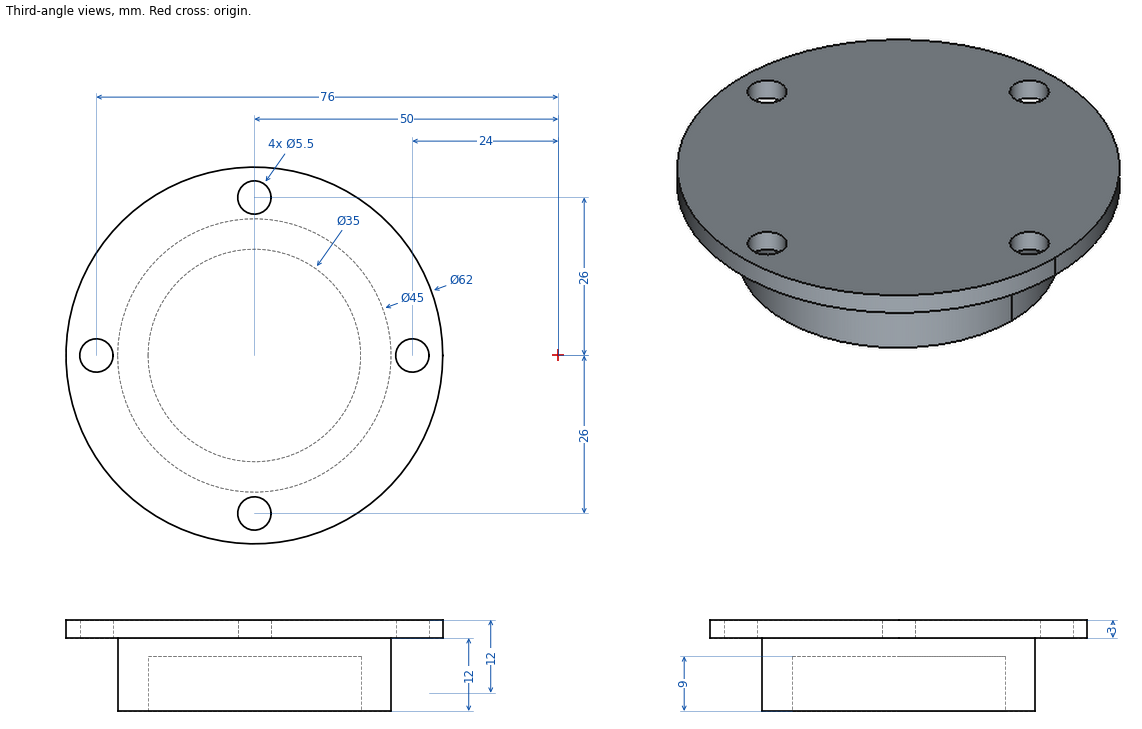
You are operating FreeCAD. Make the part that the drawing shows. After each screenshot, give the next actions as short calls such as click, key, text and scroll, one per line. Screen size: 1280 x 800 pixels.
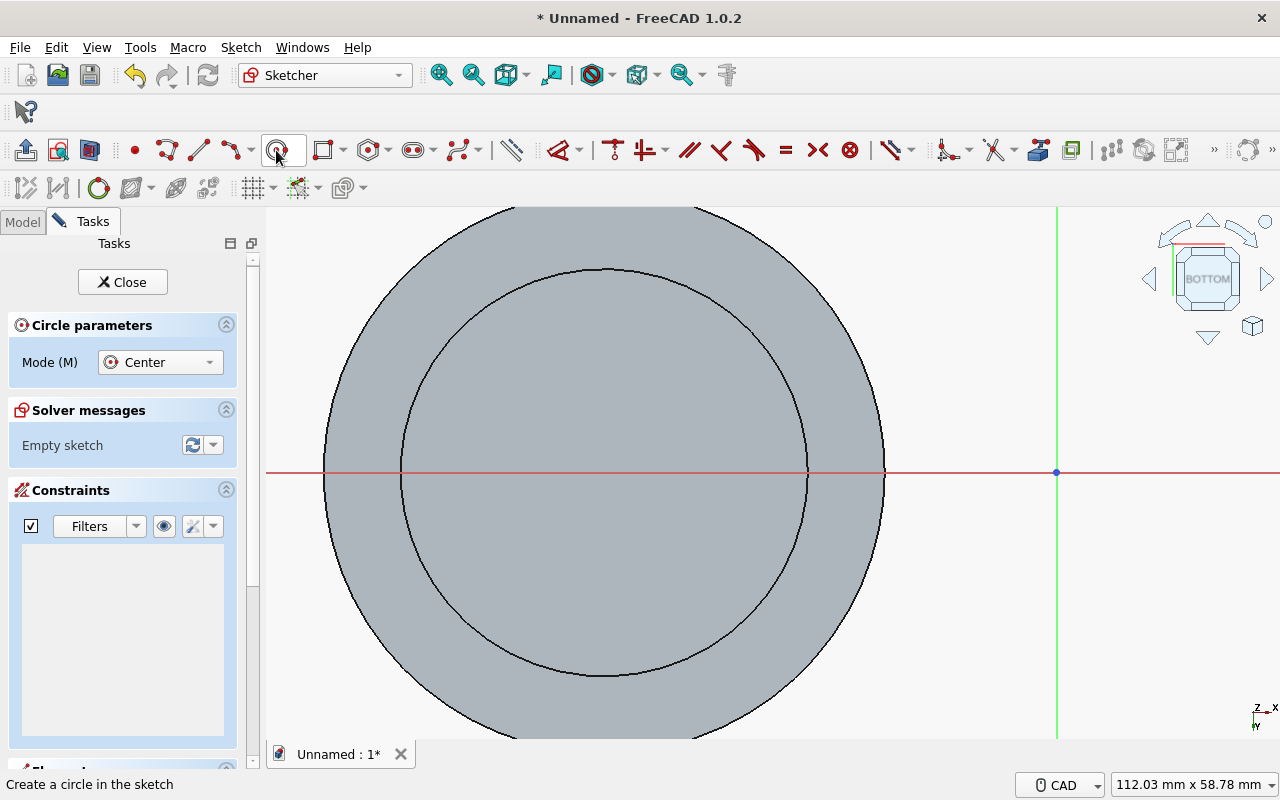
click(604, 473)
move(716, 361)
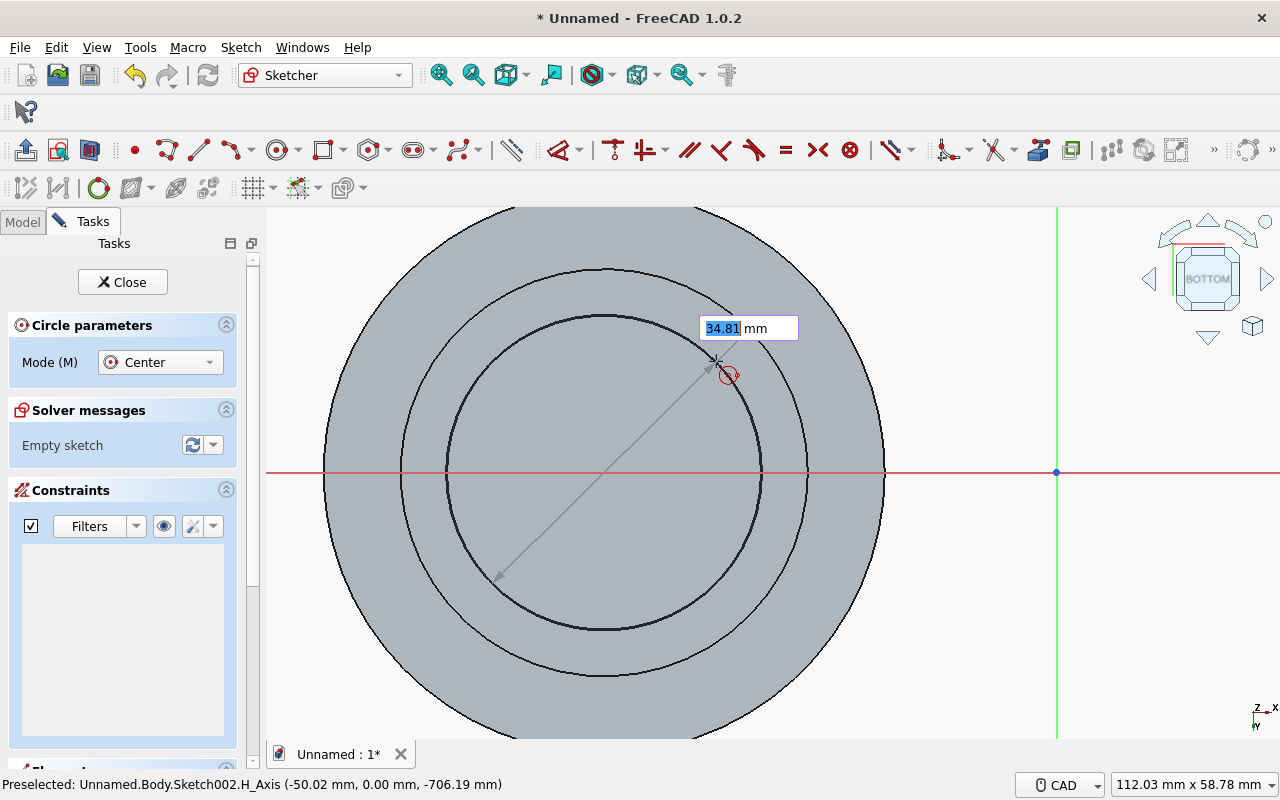
text(35)
key(Return)
key(Escape)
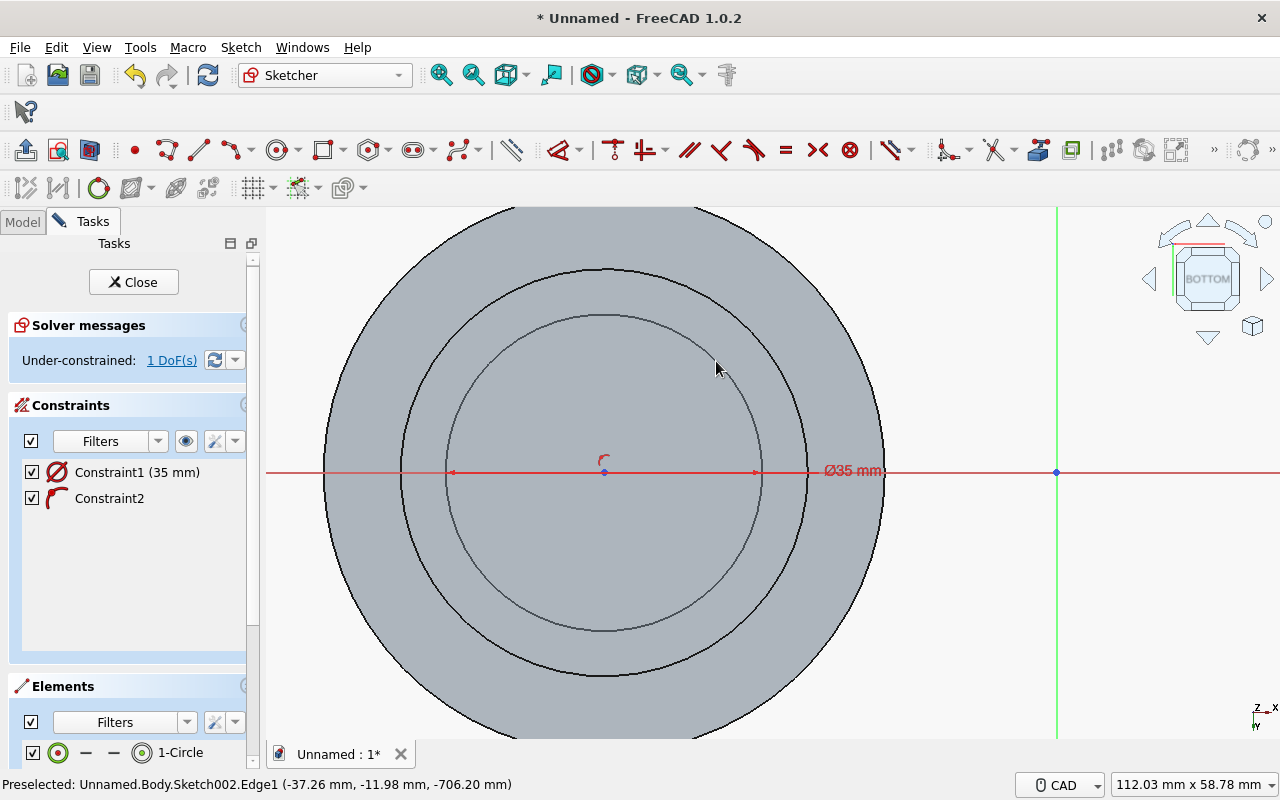
click(558, 150)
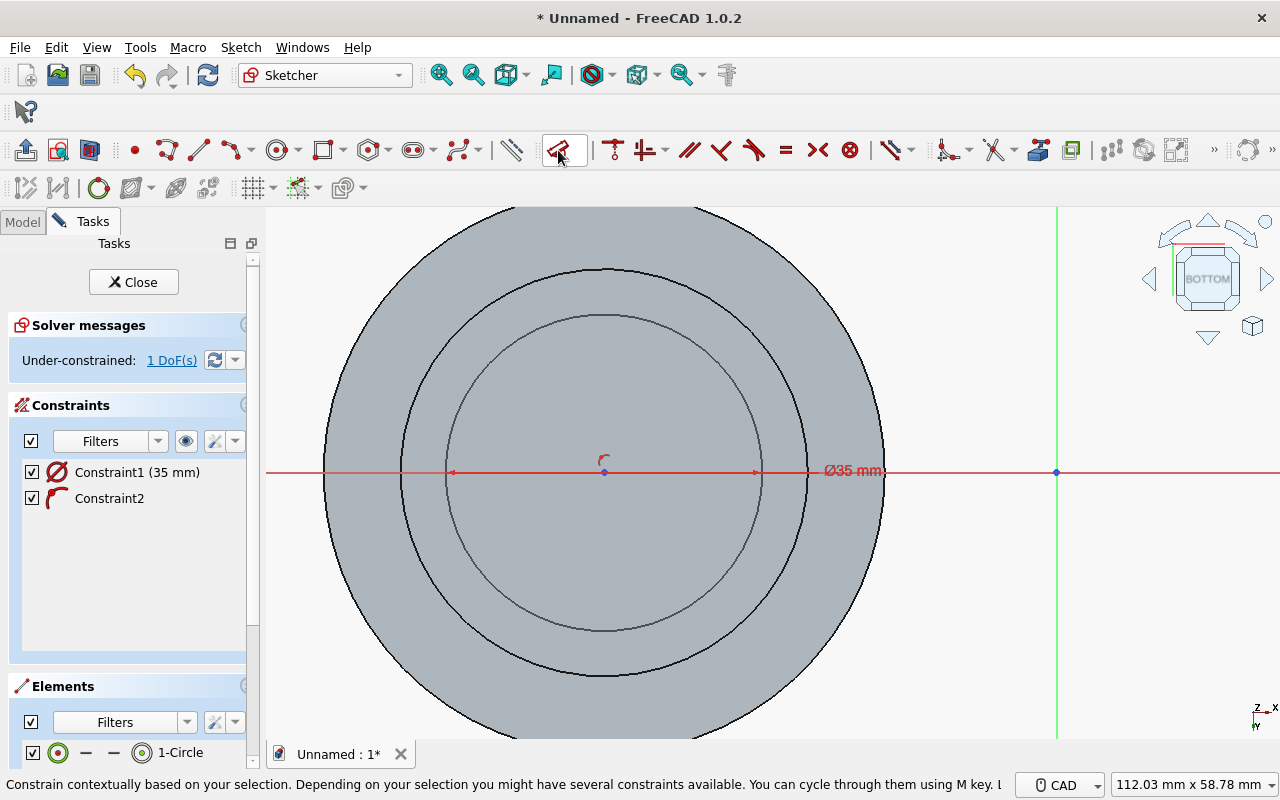
click(604, 473)
click(830, 507)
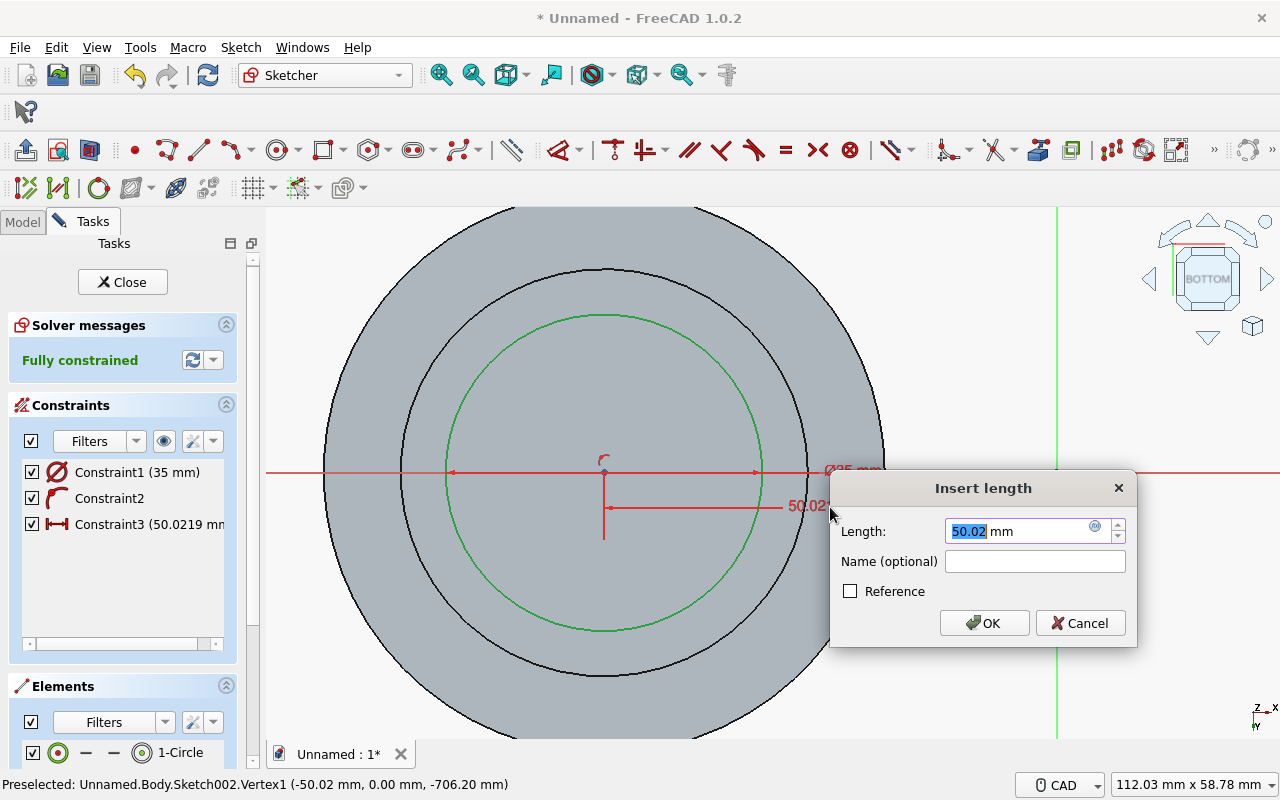
text(50)
key(Return)
key(Escape)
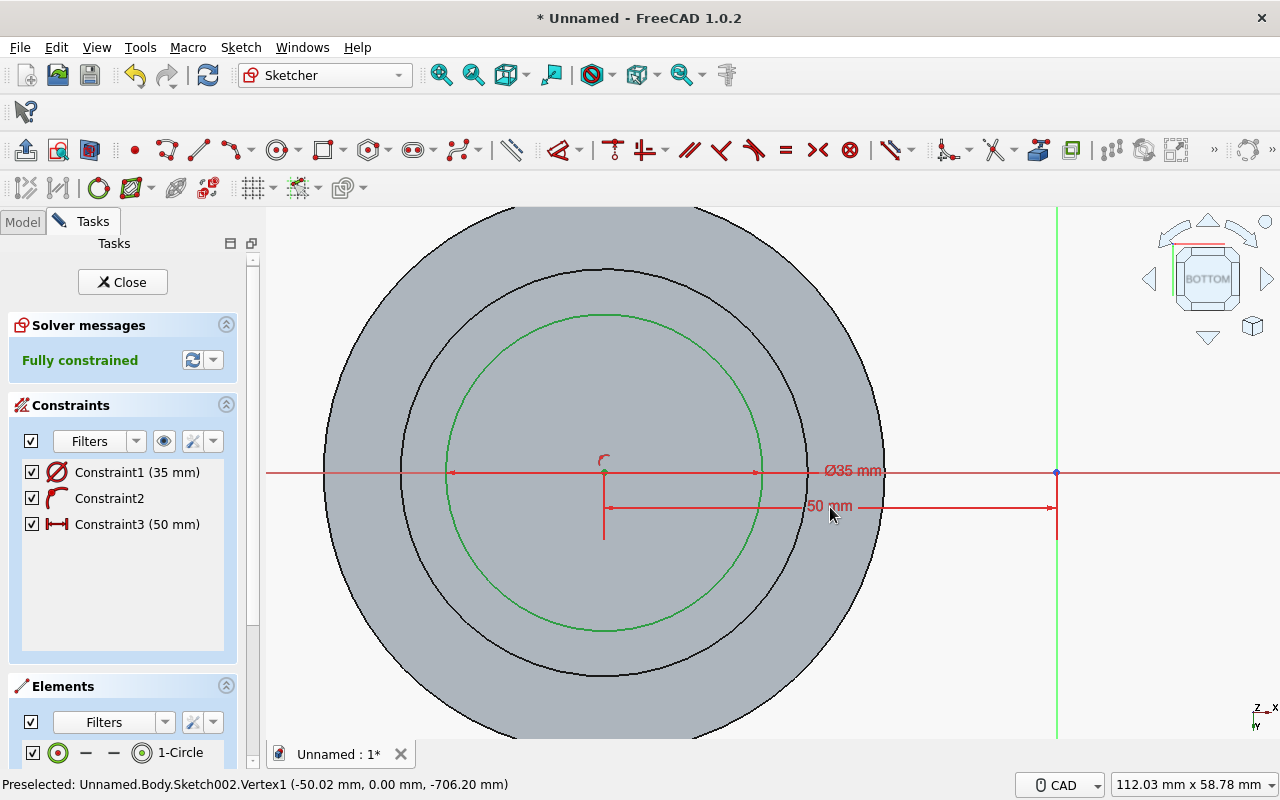
click(123, 282)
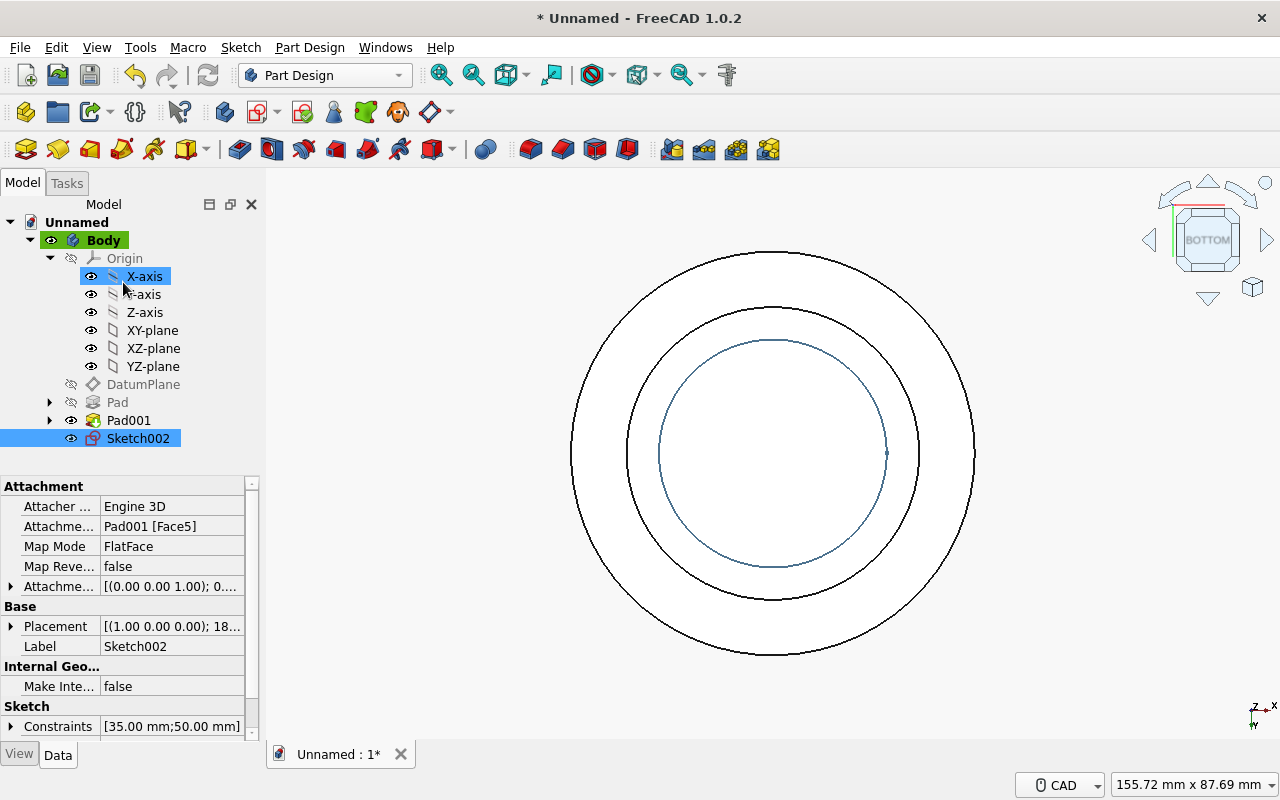
click(240, 150)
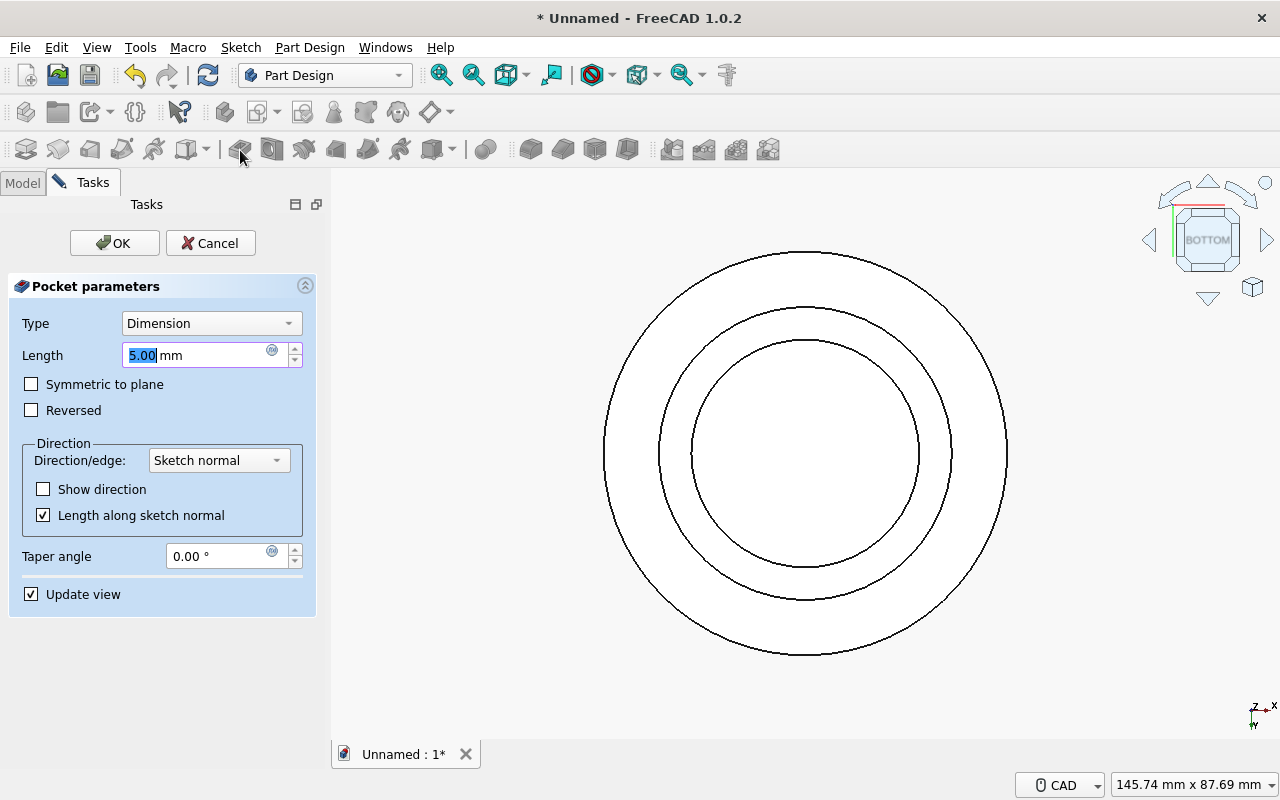
text(9)
key(Tab)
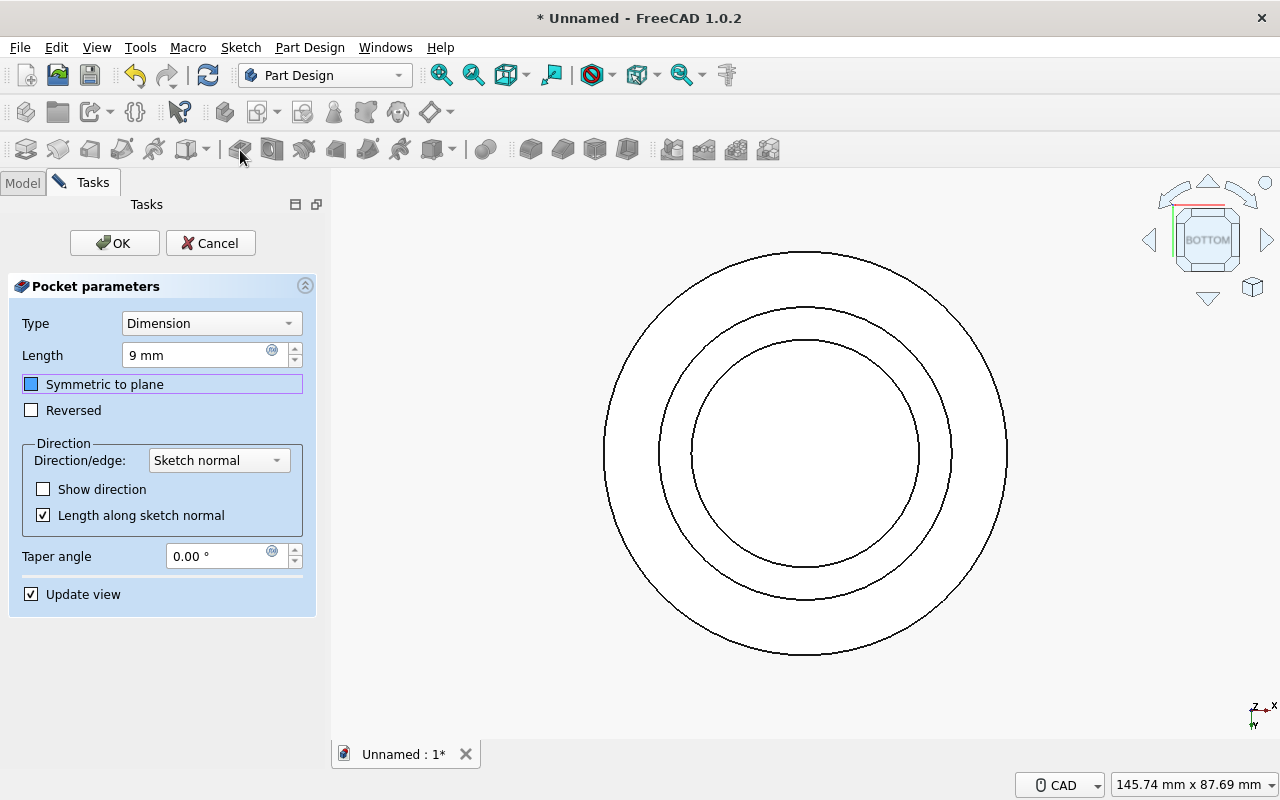
click(115, 243)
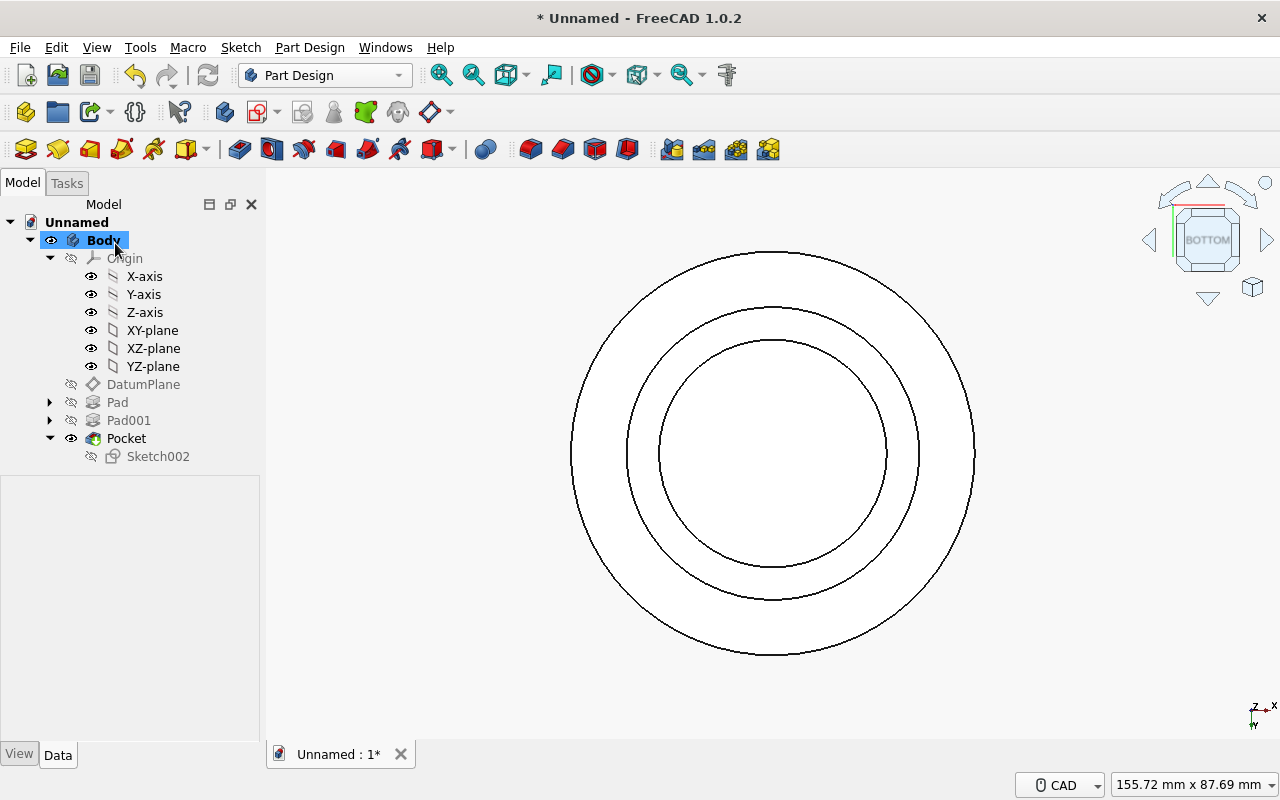
key(0)